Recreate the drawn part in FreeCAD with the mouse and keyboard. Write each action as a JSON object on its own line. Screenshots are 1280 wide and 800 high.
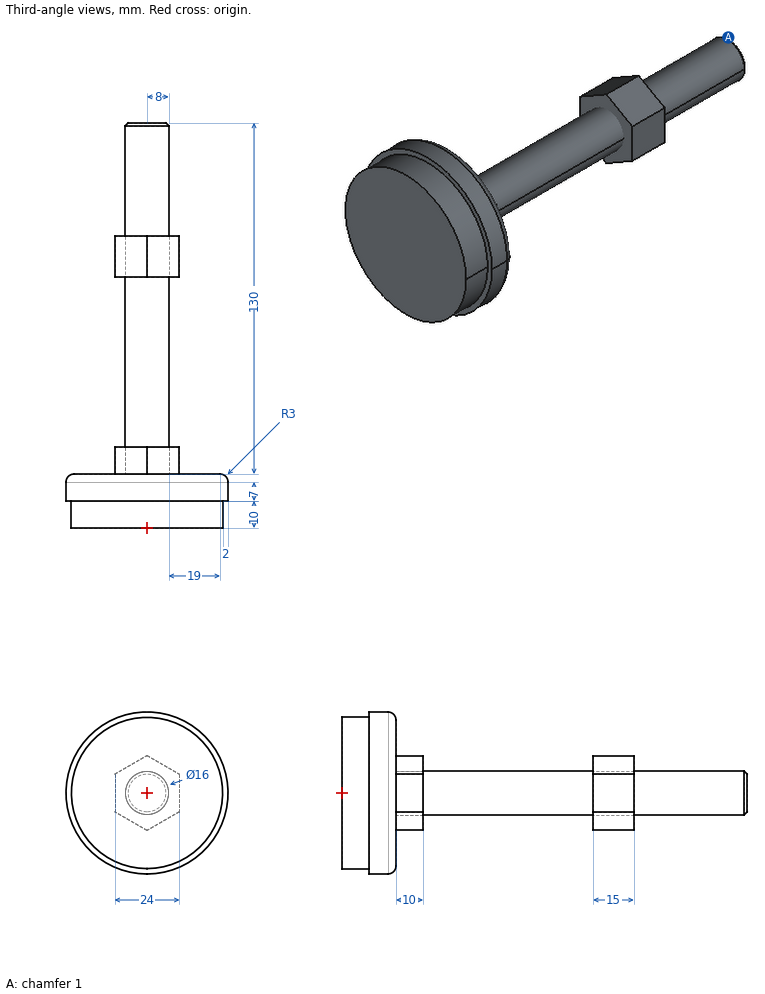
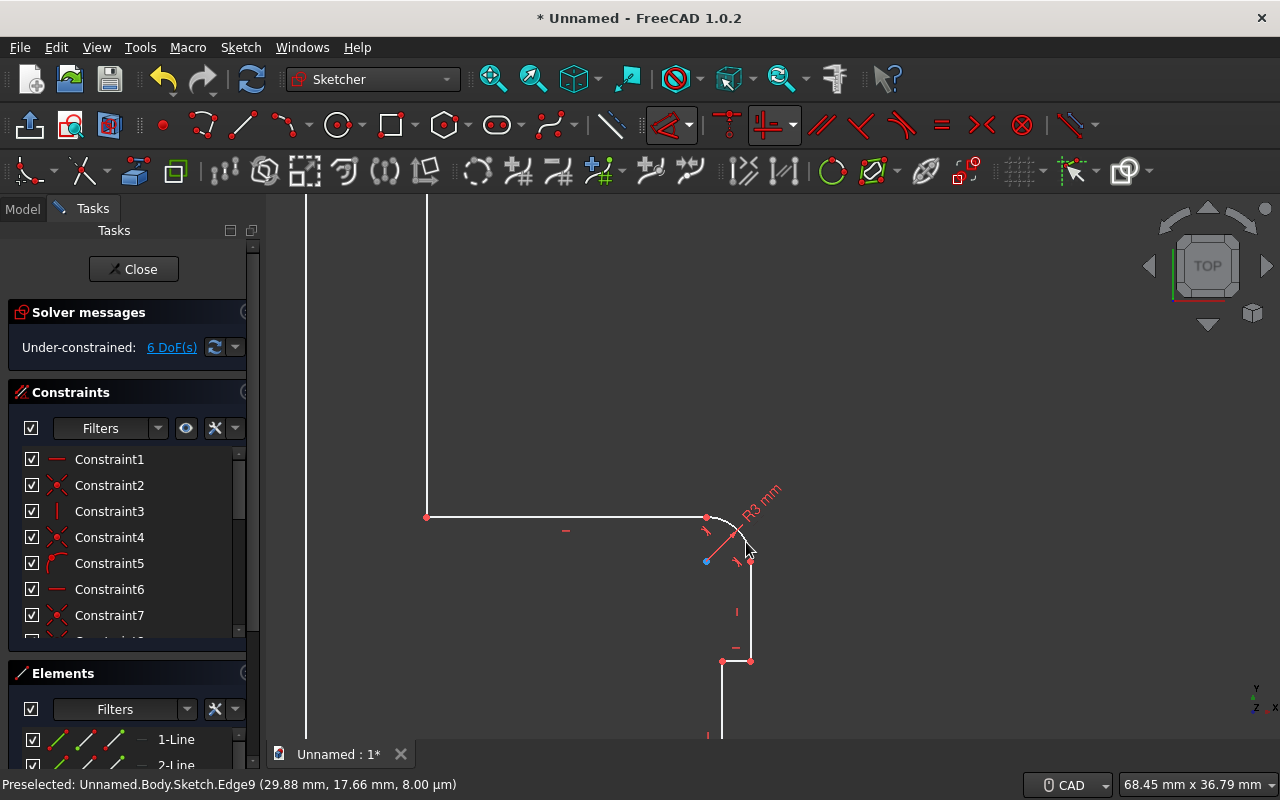
{"action": "scroll", "coordinate": [739, 619], "scroll_direction": "down", "scroll_amount": 9}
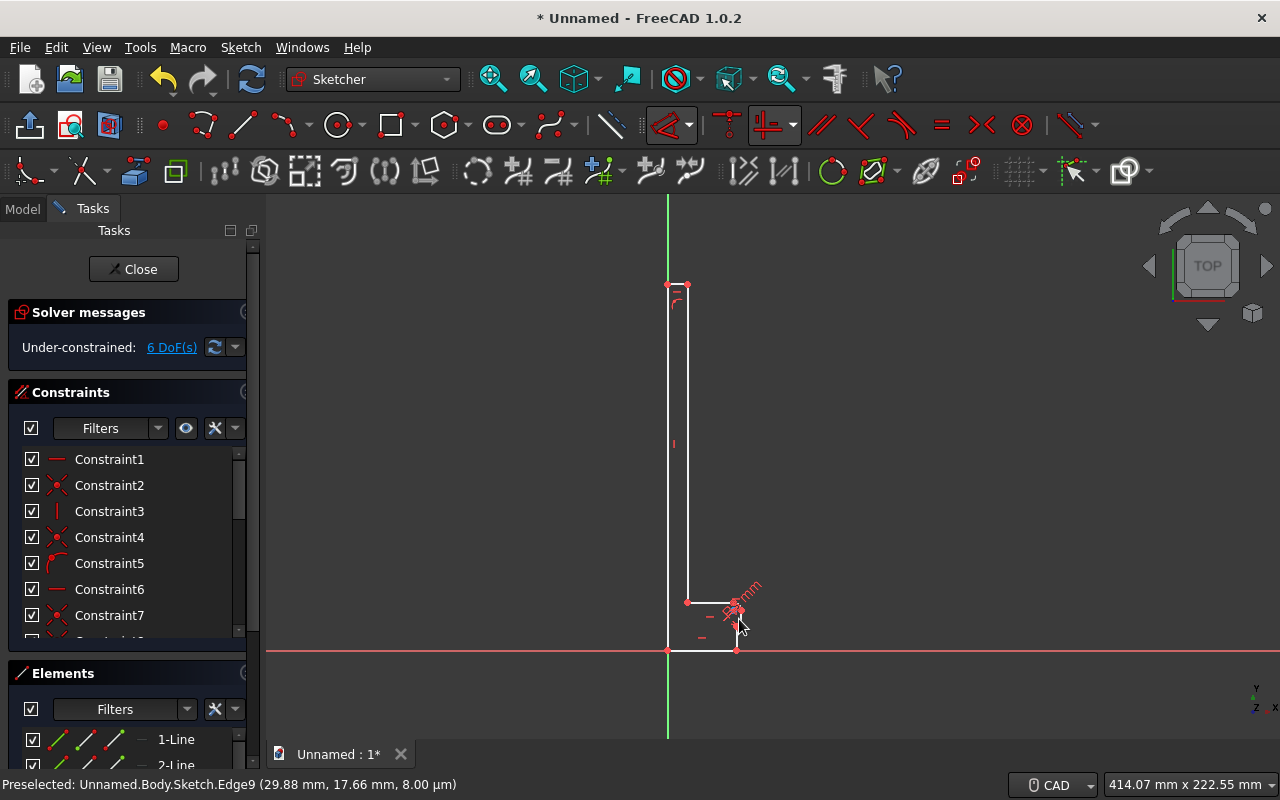
{"action": "scroll", "coordinate": [682, 284], "scroll_direction": "up", "scroll_amount": 5}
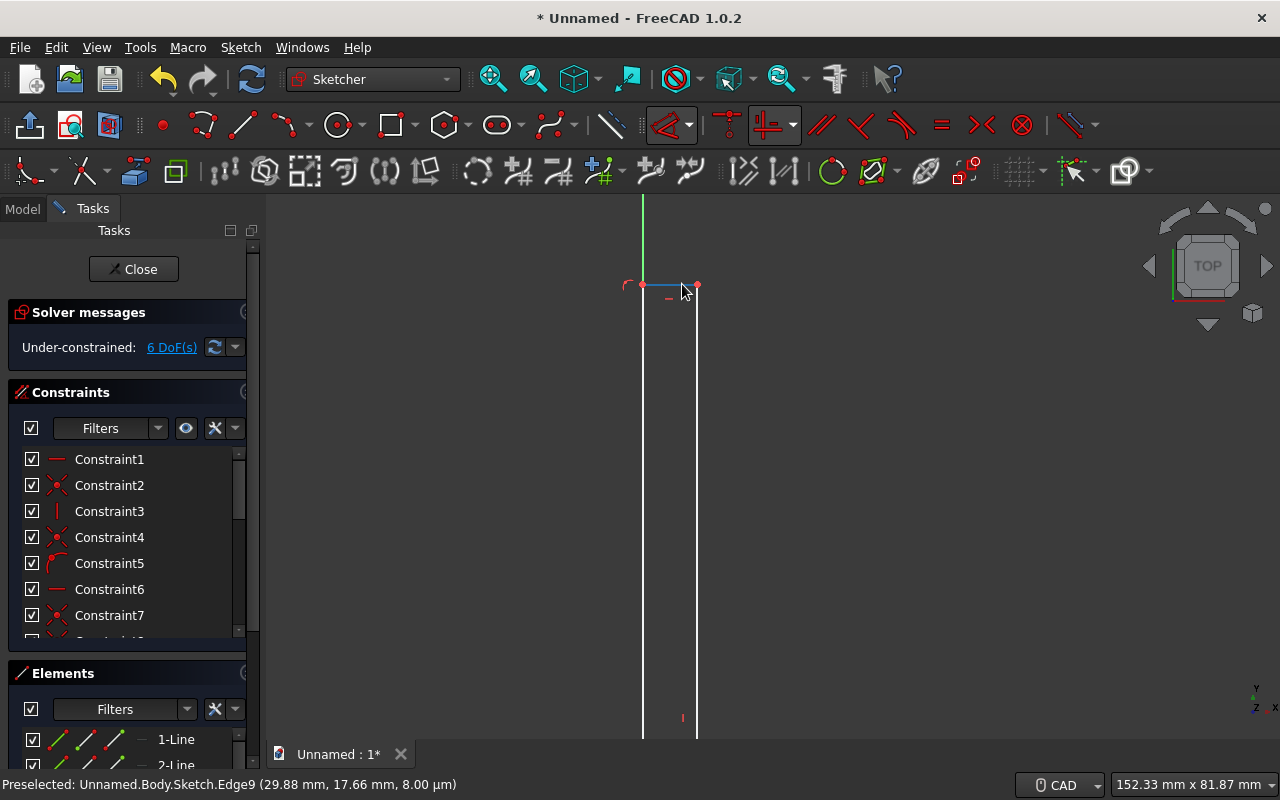
{"action": "left_click", "coordinate": [681, 285]}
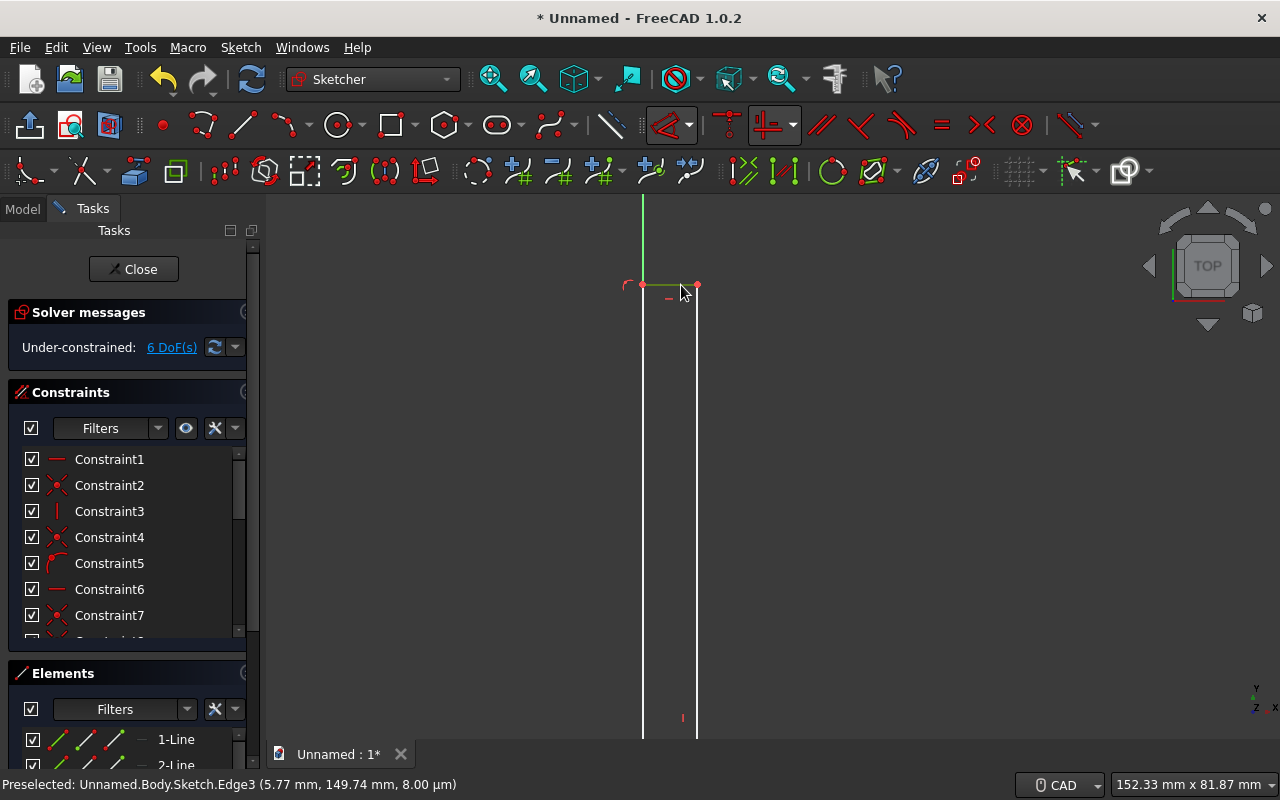
{"action": "key", "text": "l"}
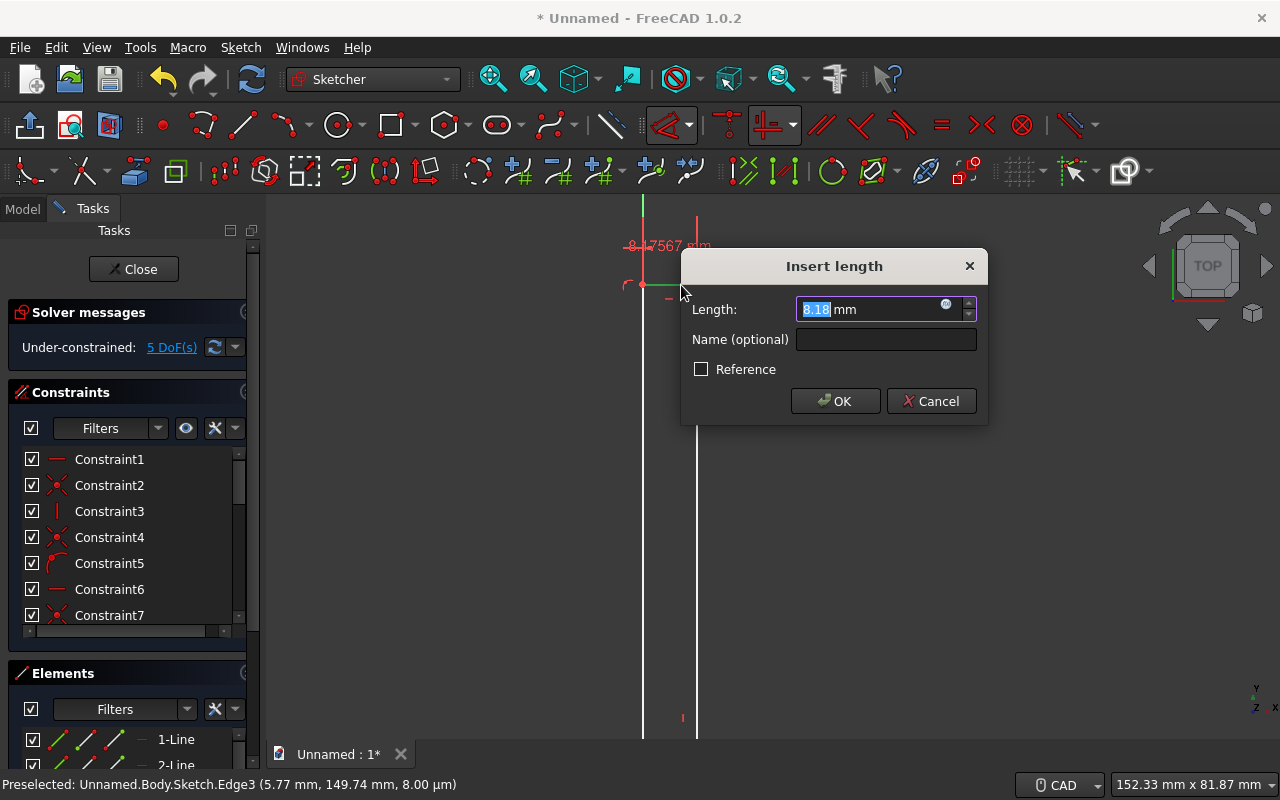
{"action": "type", "text": "8"}
{"action": "key", "text": "Return"}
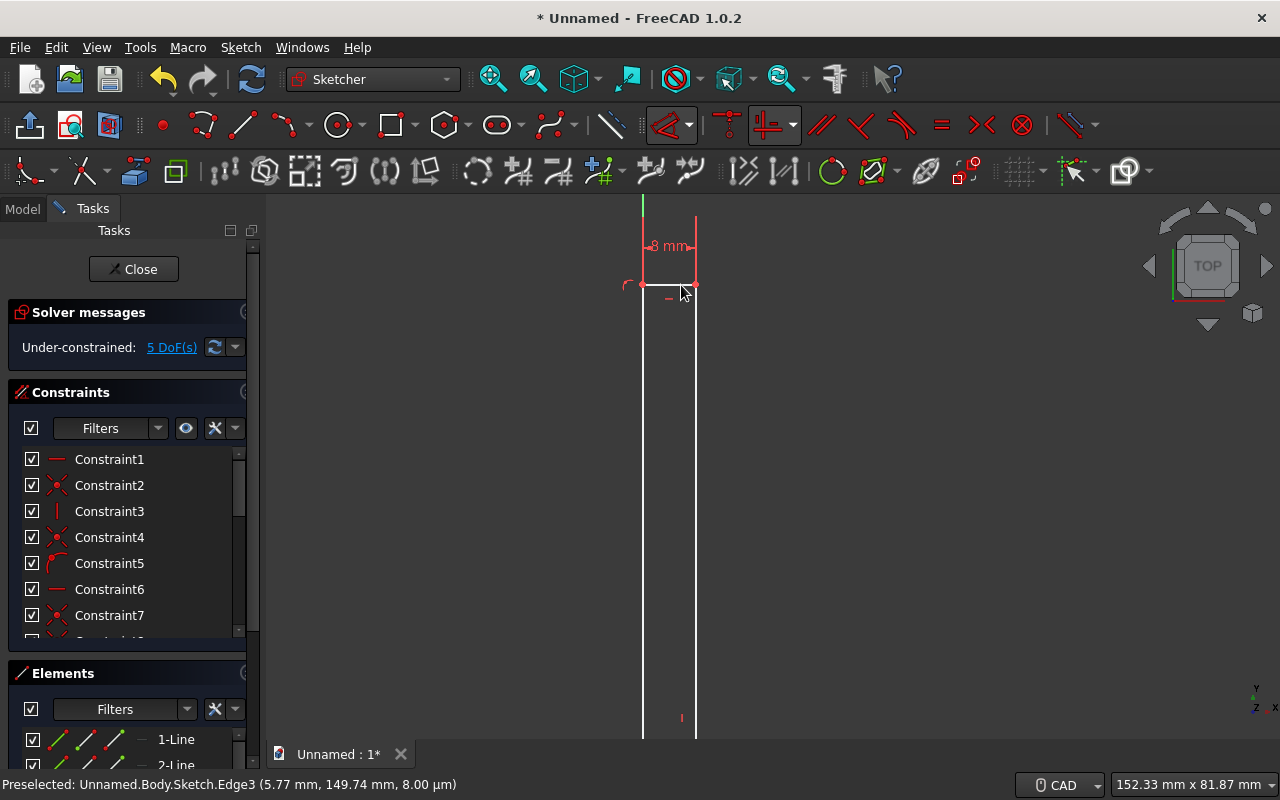
{"action": "scroll", "coordinate": [682, 283], "scroll_direction": "down", "scroll_amount": 5}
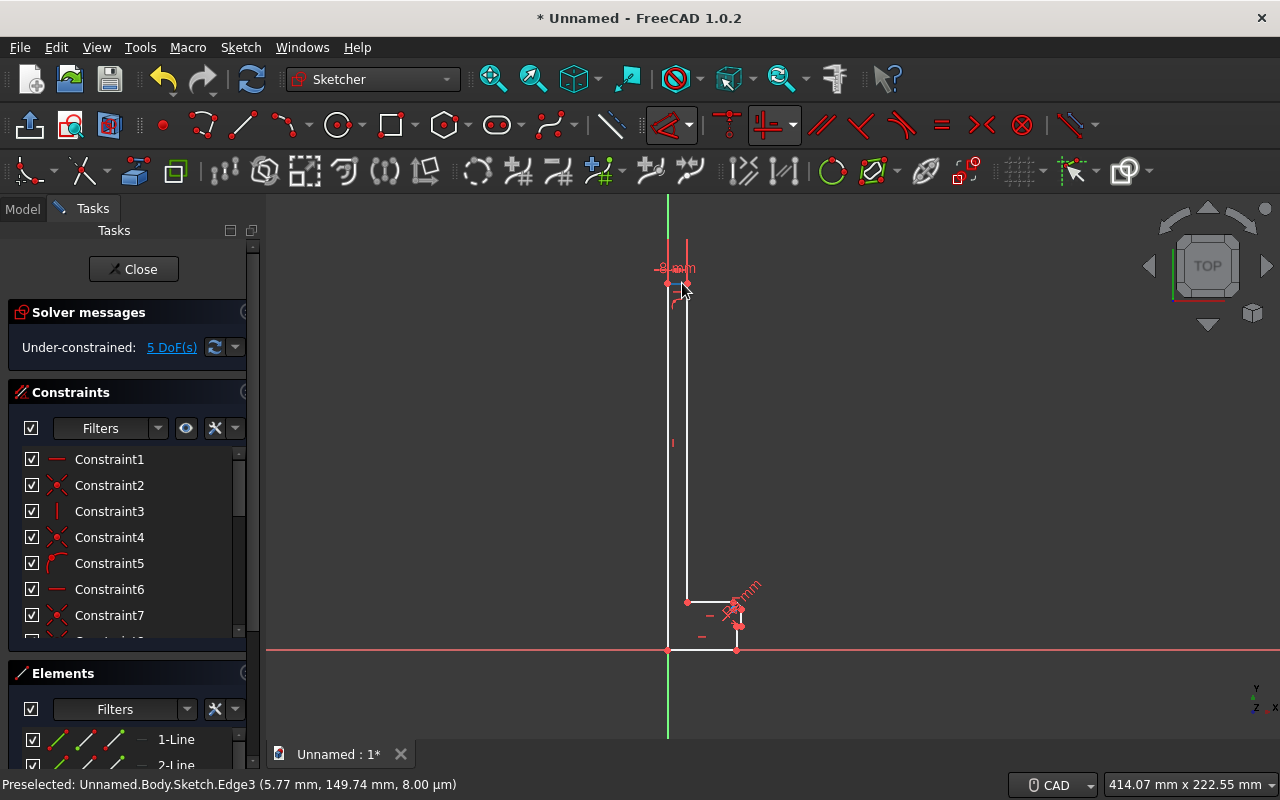
{"action": "scroll", "coordinate": [739, 626], "scroll_direction": "up", "scroll_amount": 11}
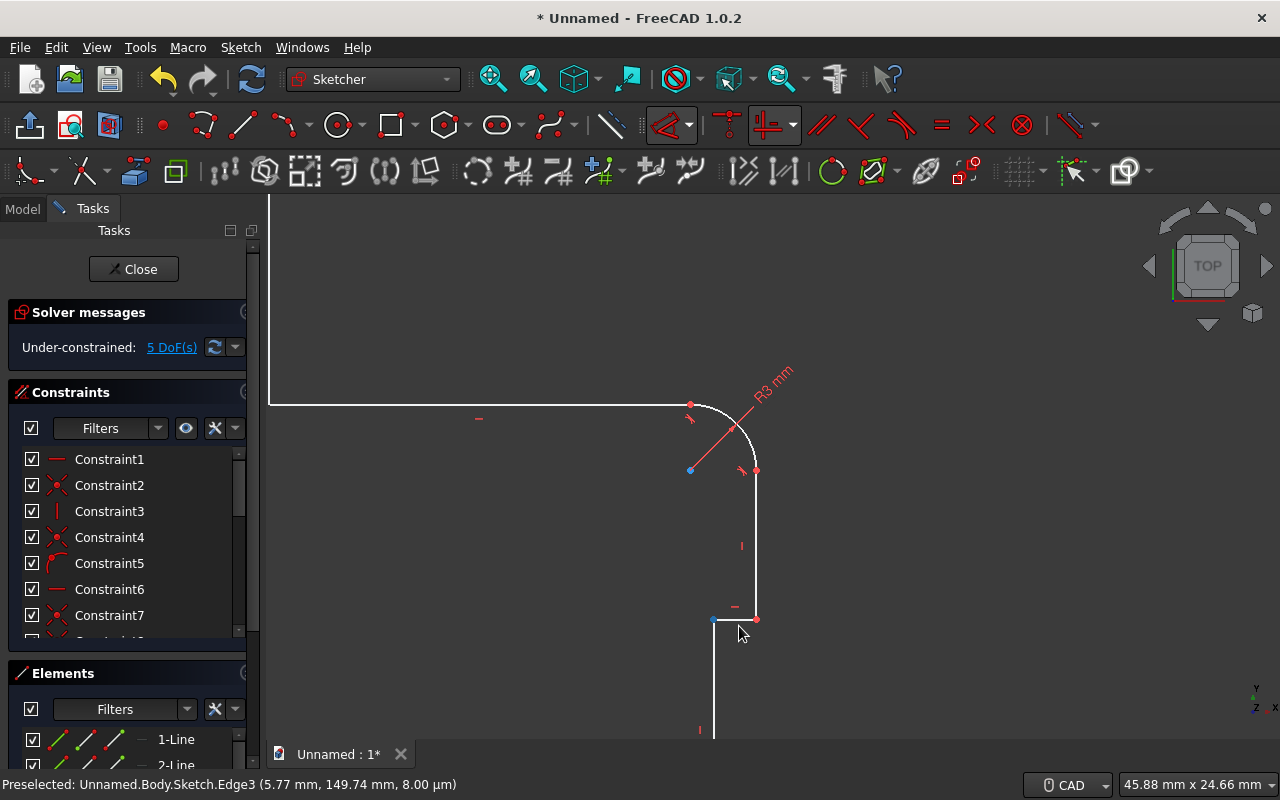
{"action": "left_click", "coordinate": [735, 620]}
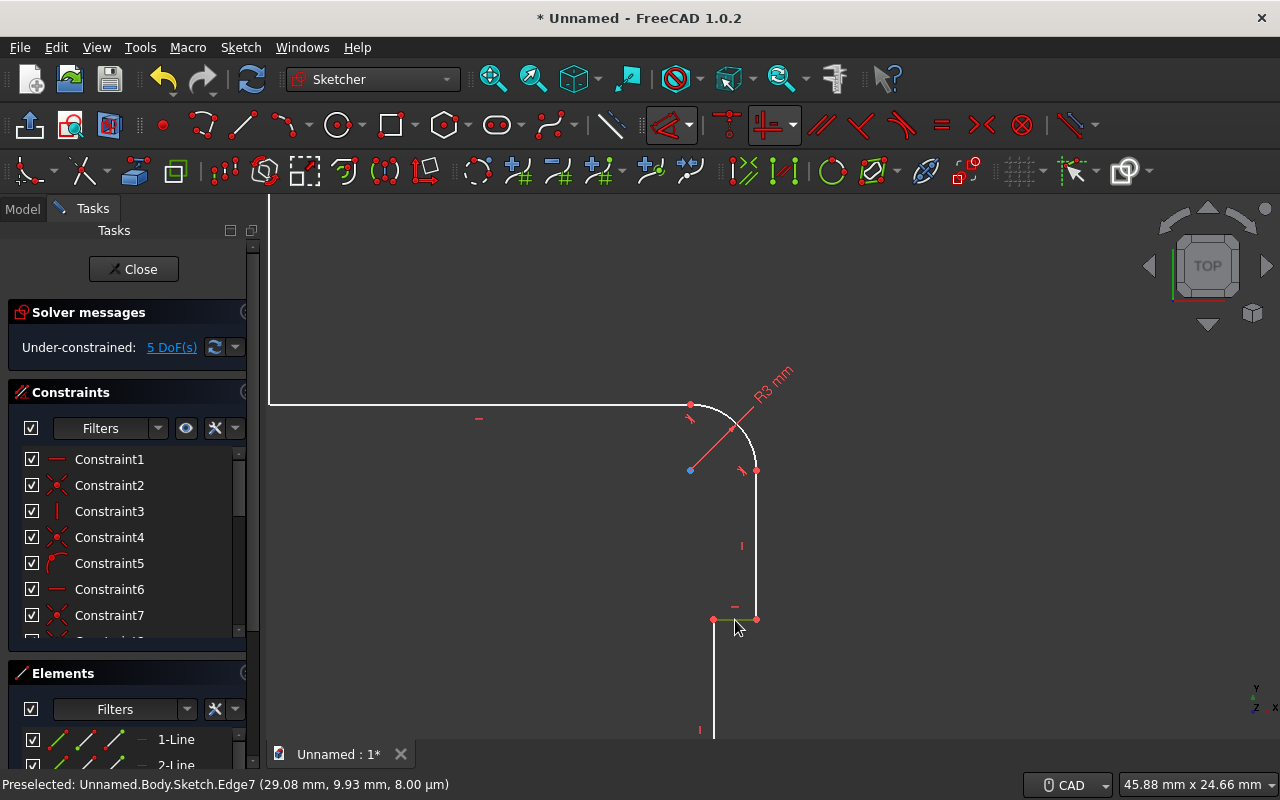
{"action": "key", "text": "l"}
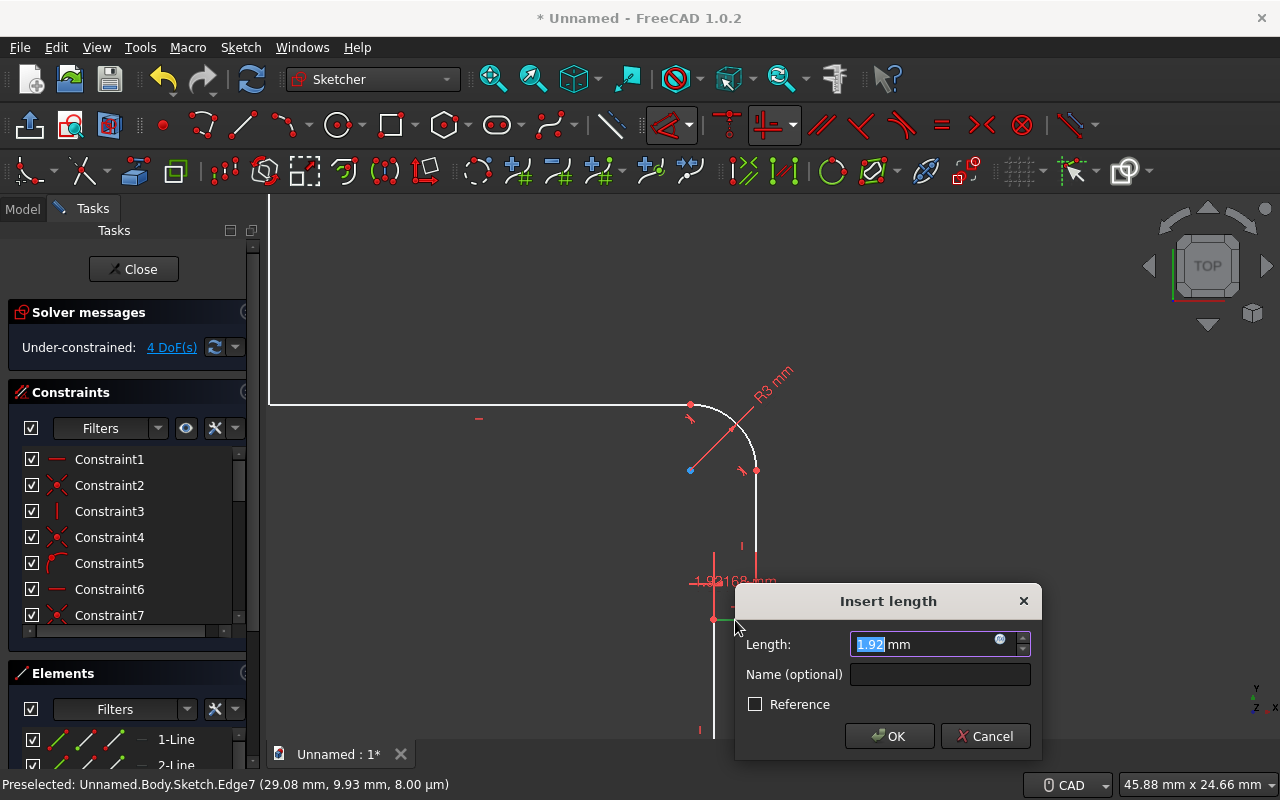
{"action": "type", "text": "2"}
{"action": "key", "text": "Return"}